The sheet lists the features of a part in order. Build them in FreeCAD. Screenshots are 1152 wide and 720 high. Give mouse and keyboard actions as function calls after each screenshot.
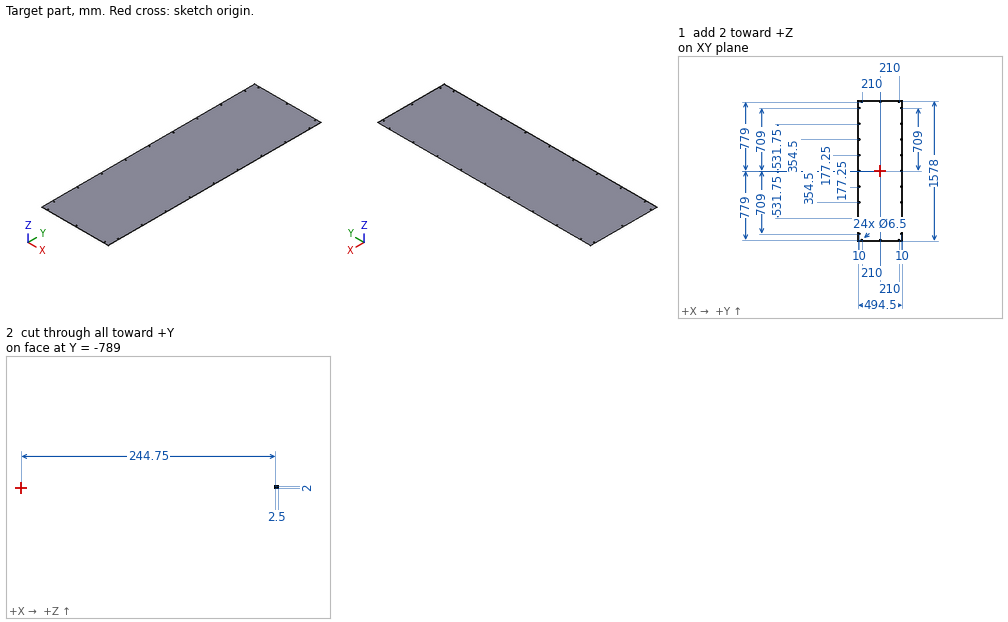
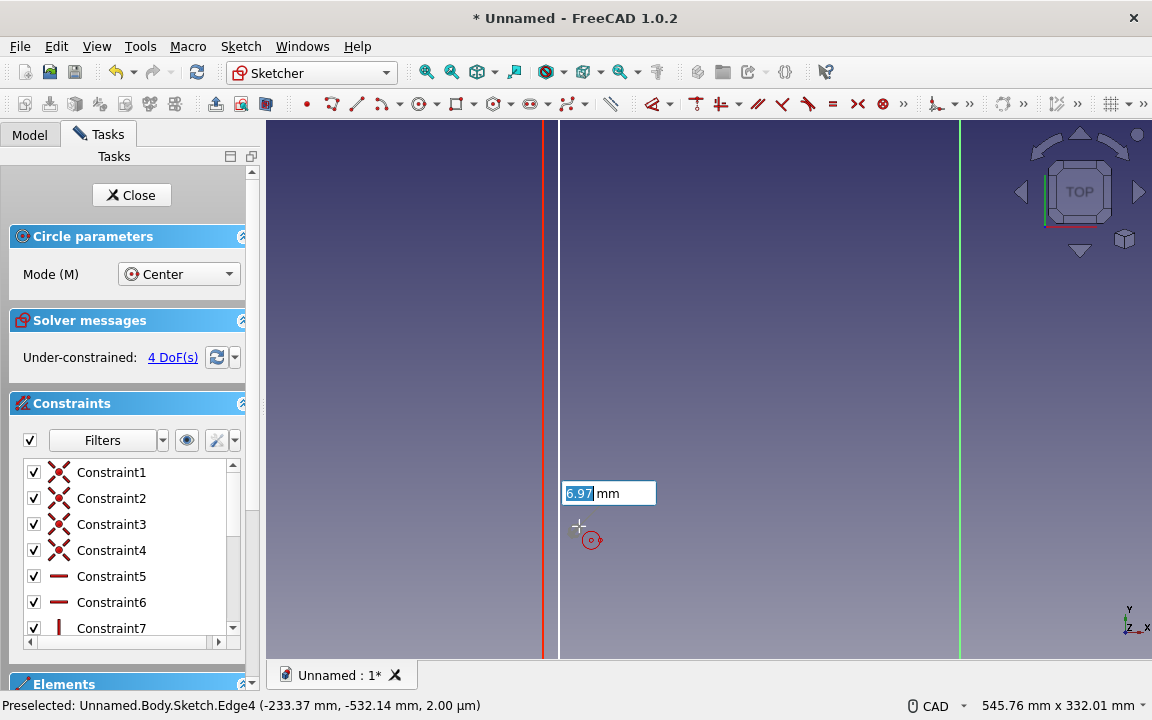
text(6.5)
key(Return)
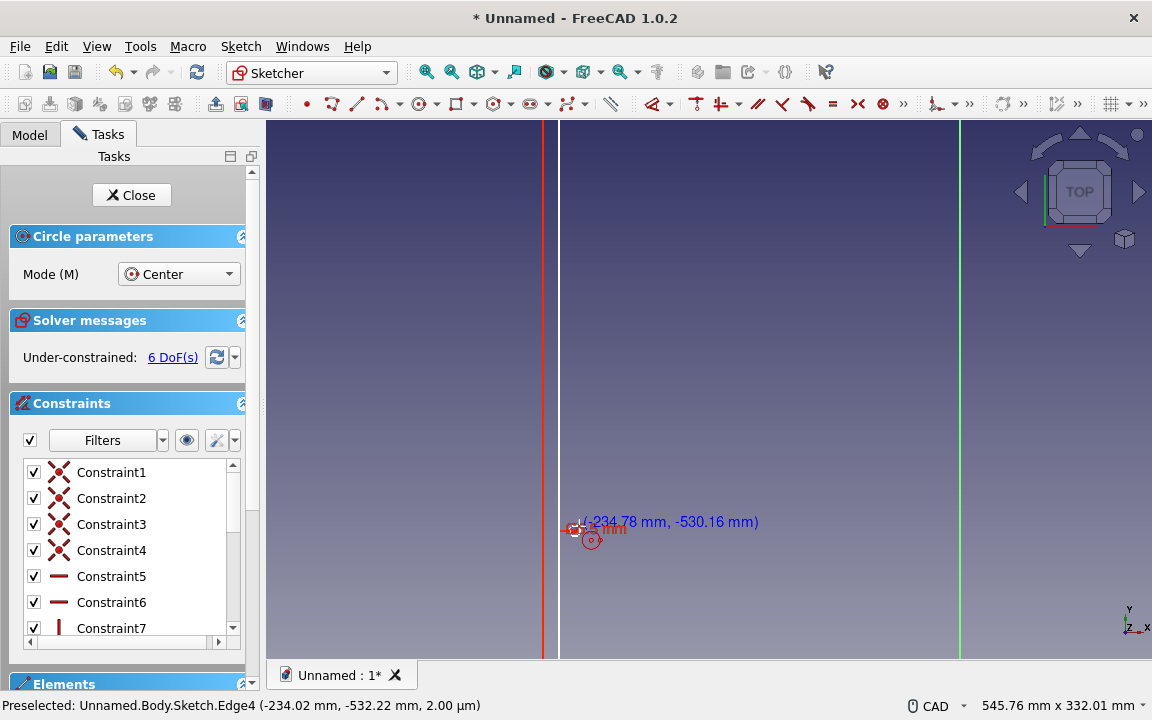
scroll(575, 242, up, 8)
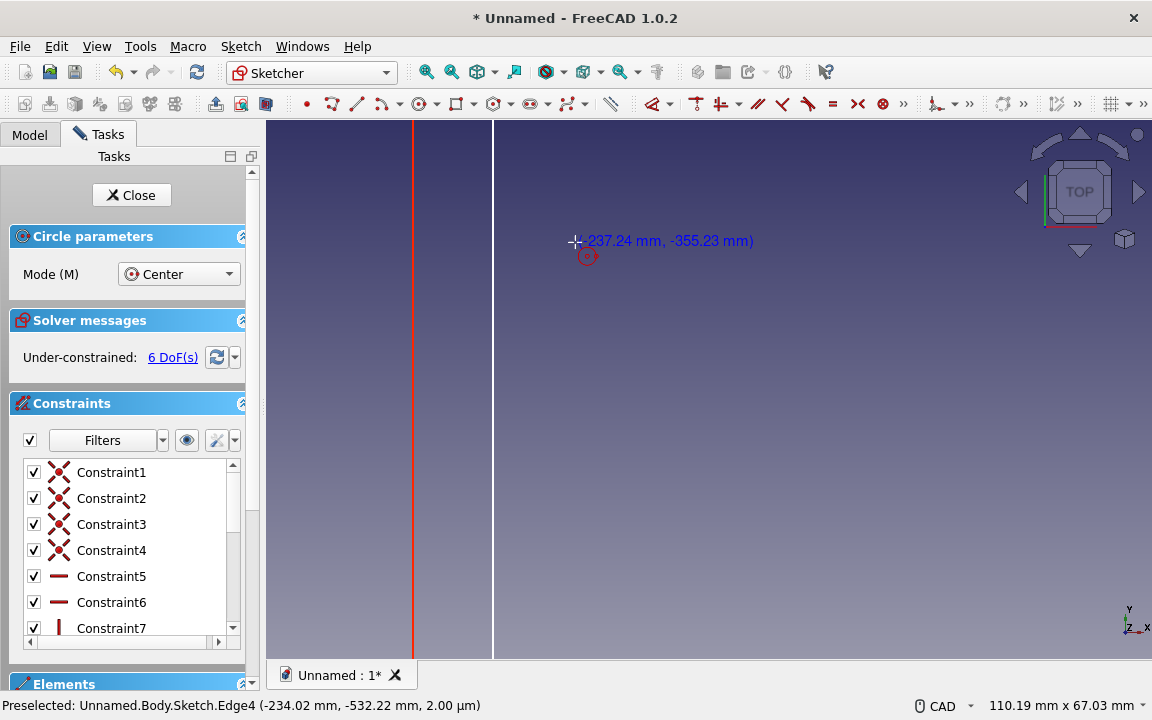
scroll(577, 493, down, 17)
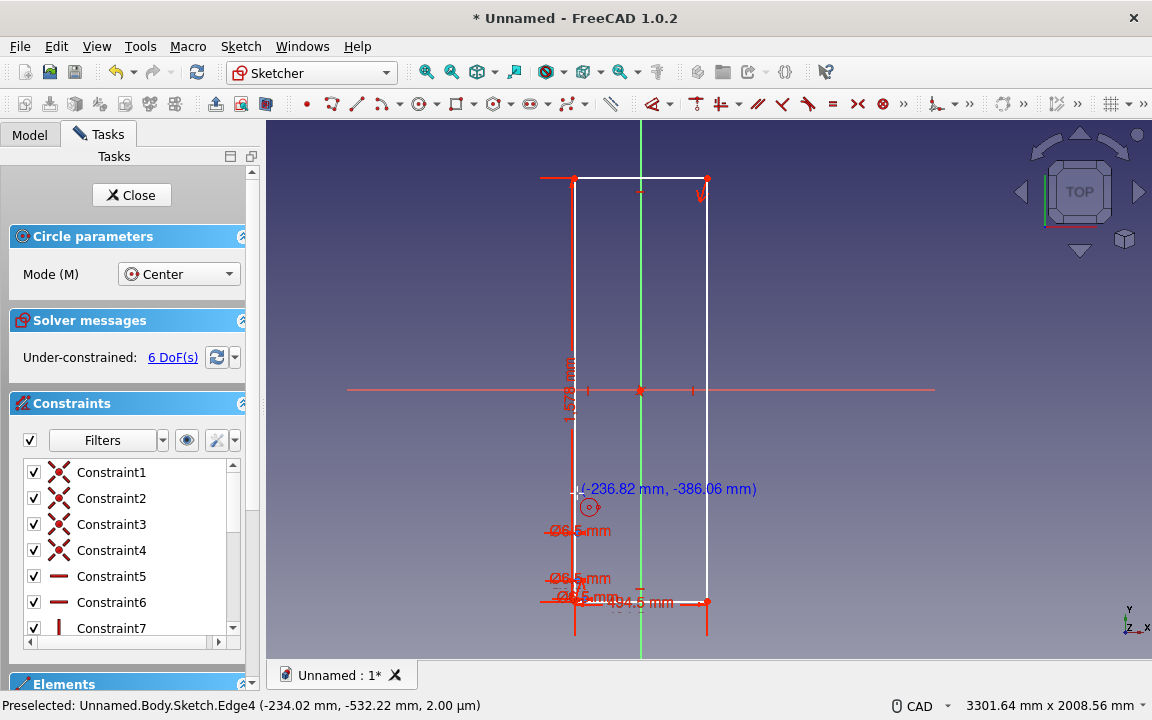
scroll(577, 485, up, 9)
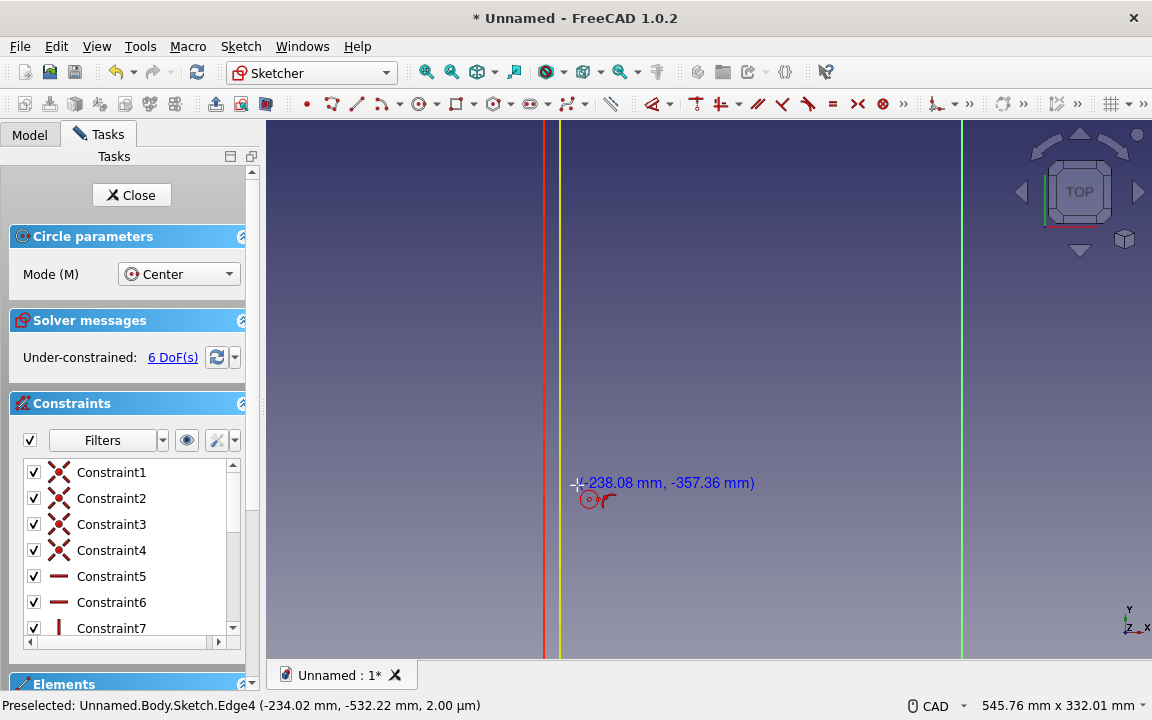
click(577, 483)
move(580, 479)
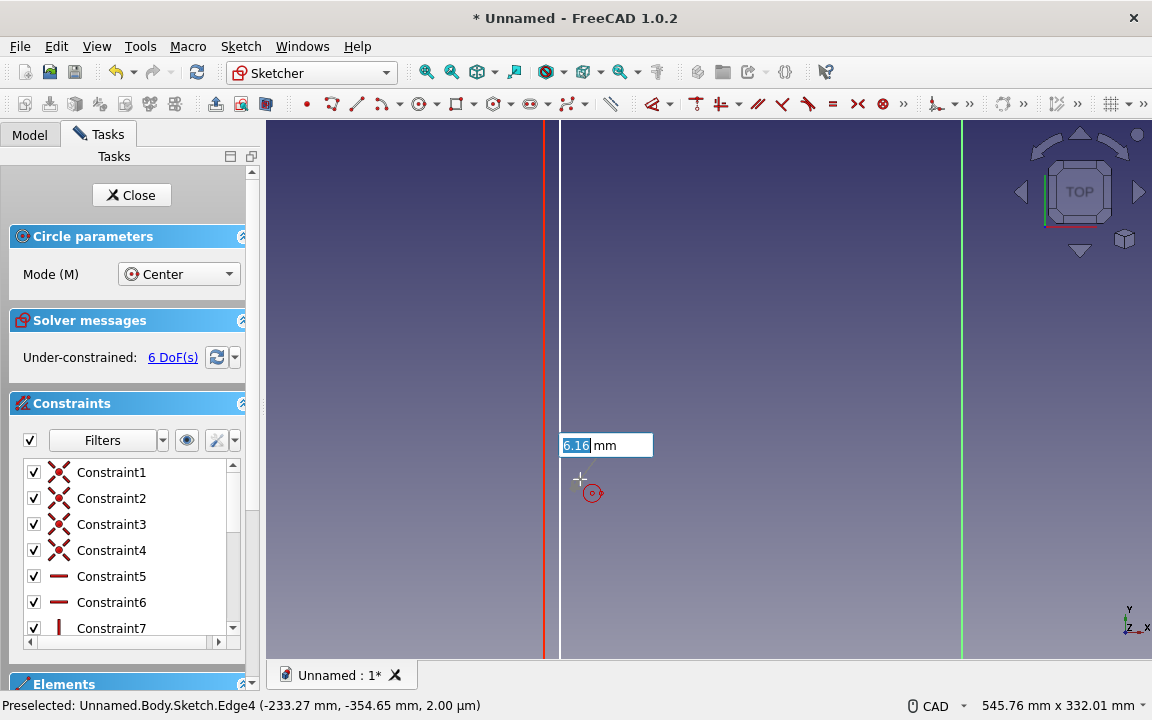
text(6.5)
key(Return)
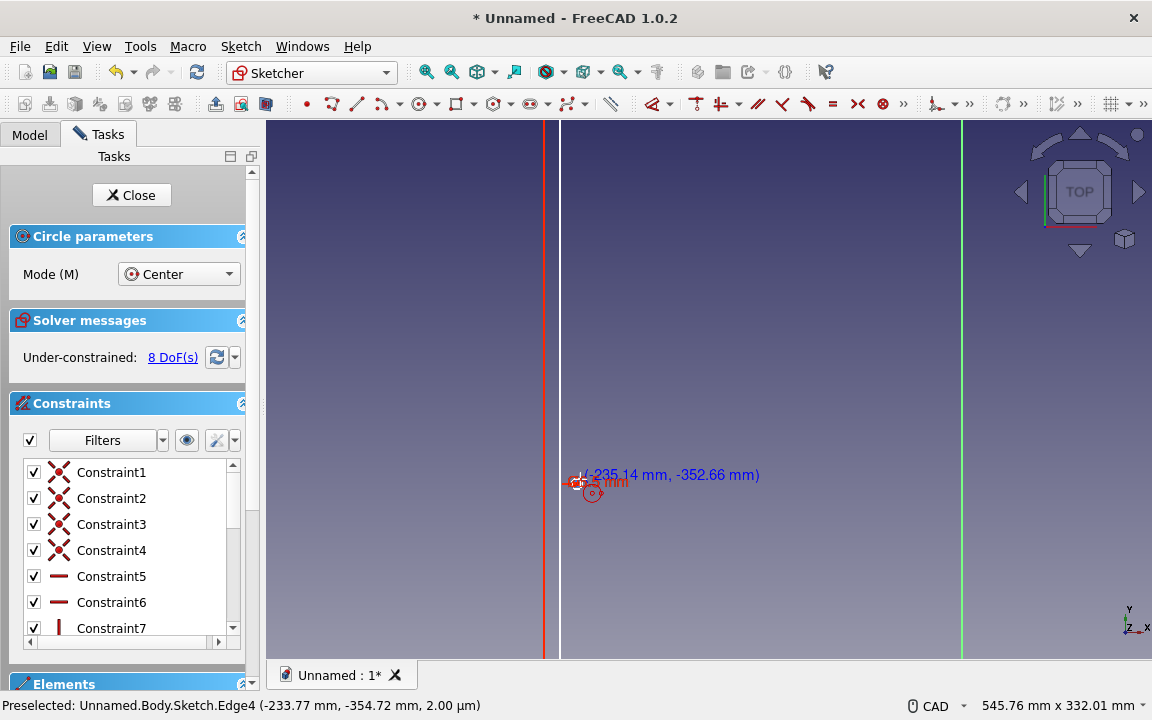
scroll(577, 195, up, 8)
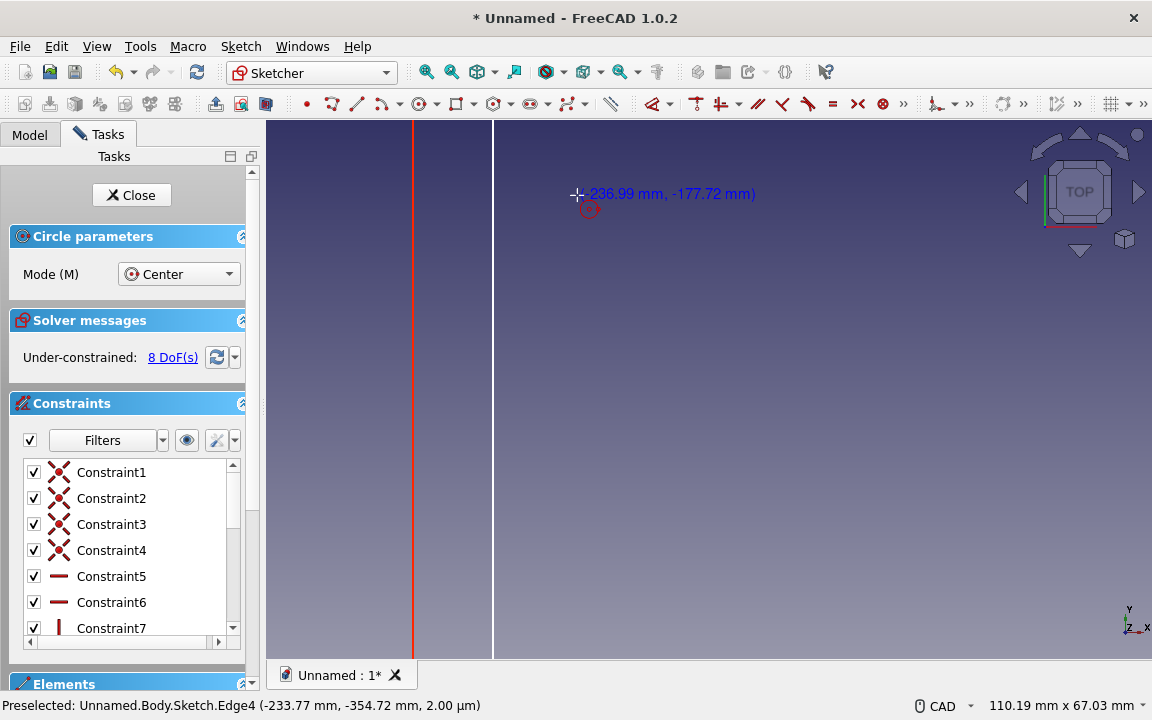
scroll(577, 445, down, 17)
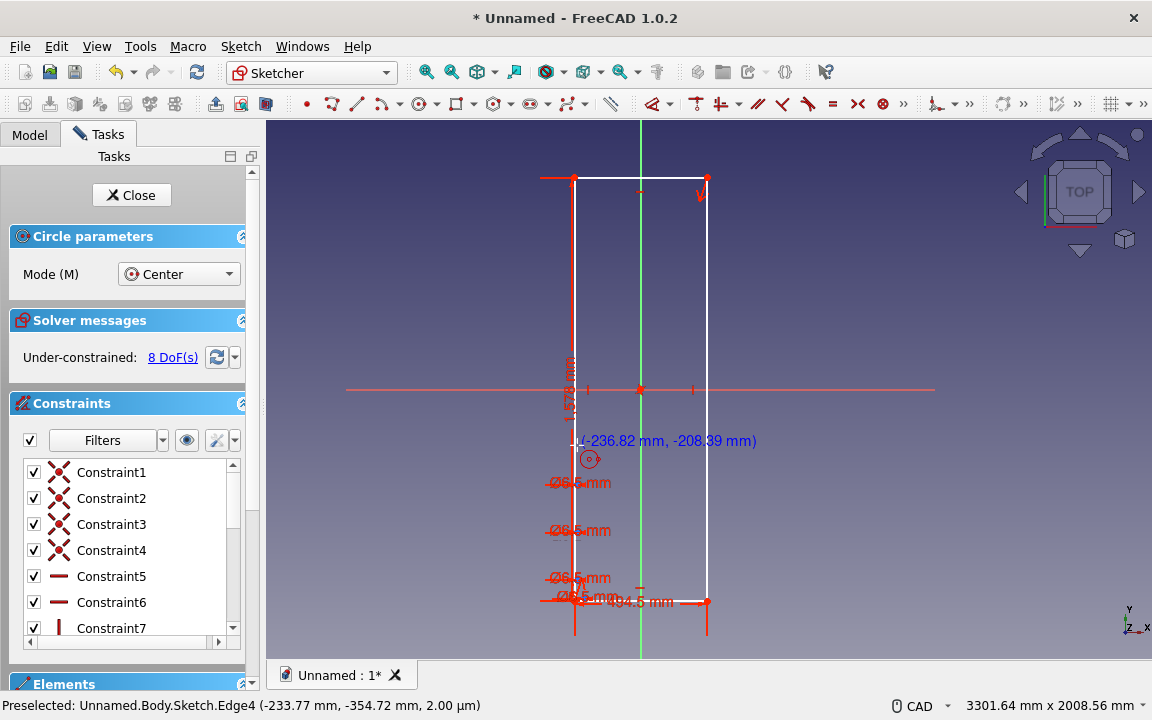
scroll(577, 437, up, 9)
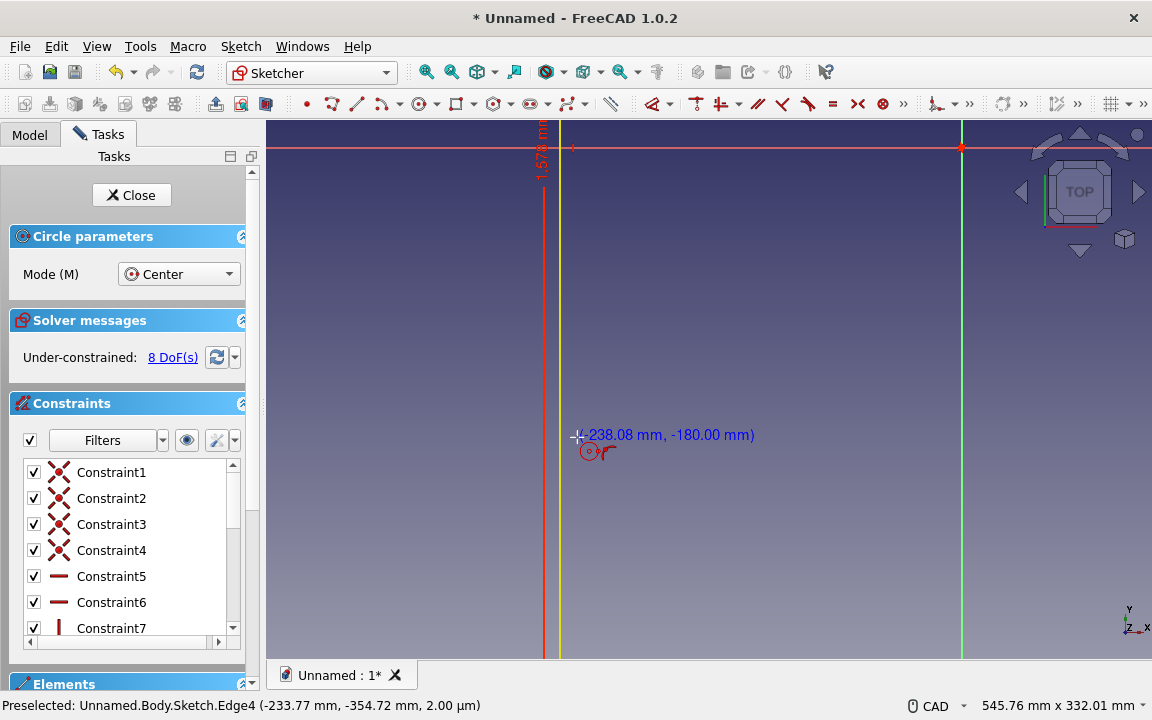
click(577, 436)
move(580, 432)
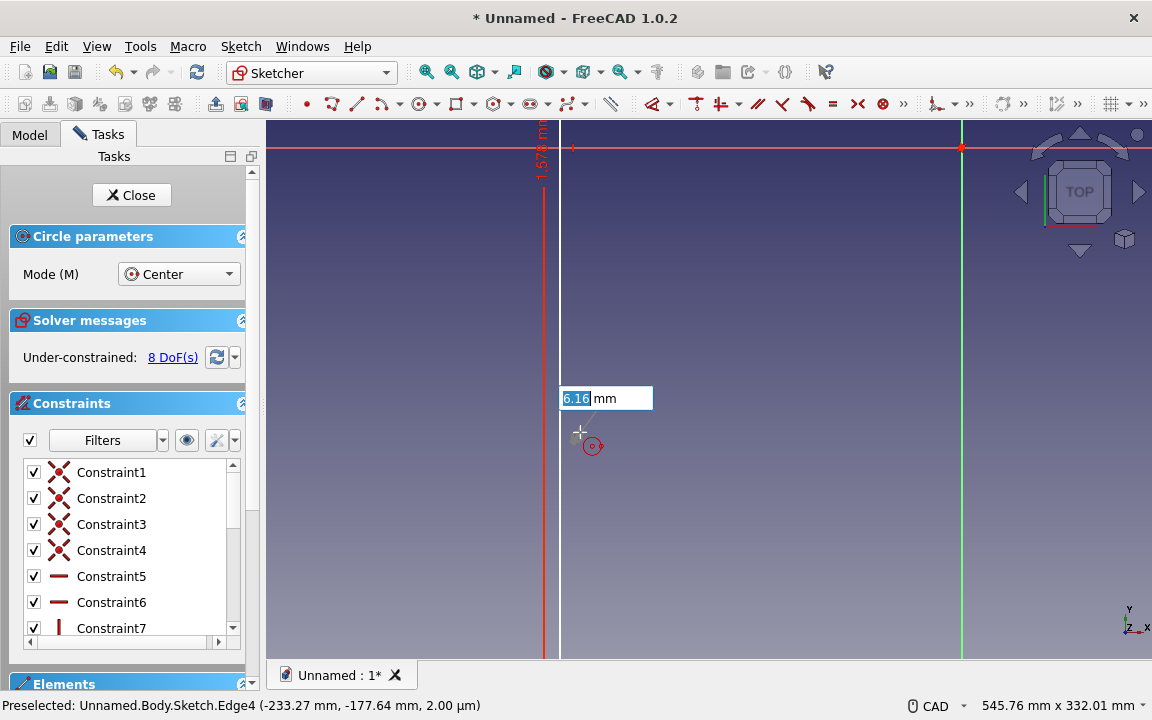
text(6.5)
key(Return)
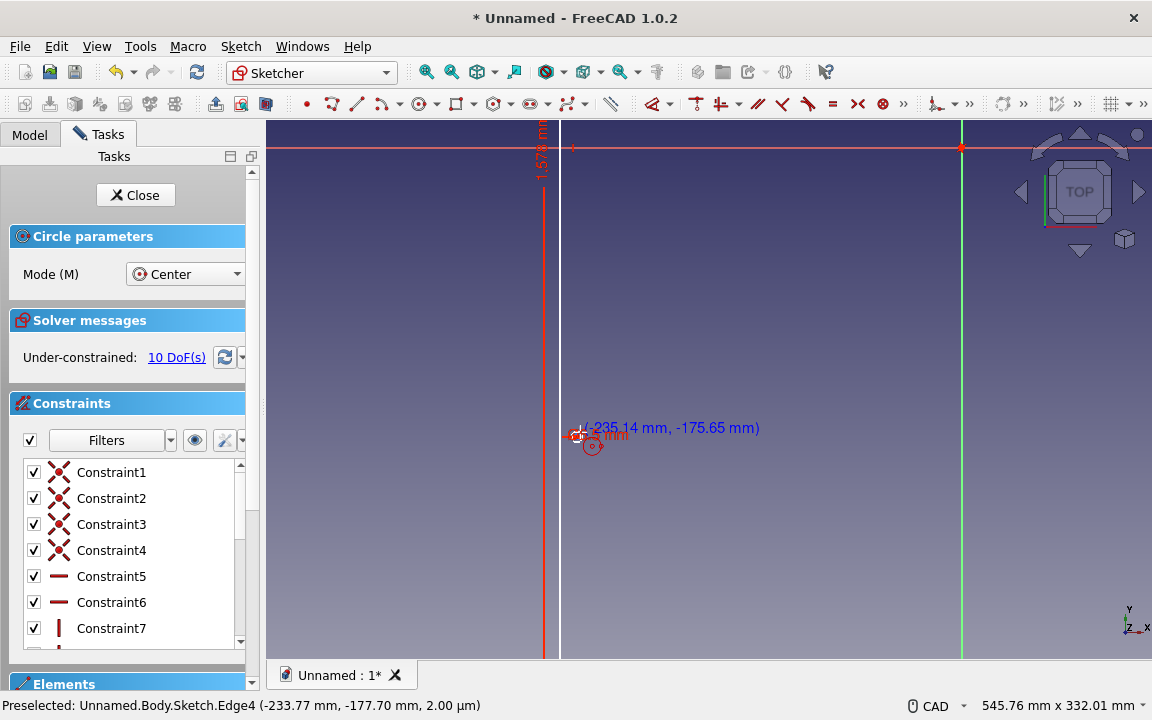
scroll(590, 427, down, 10)